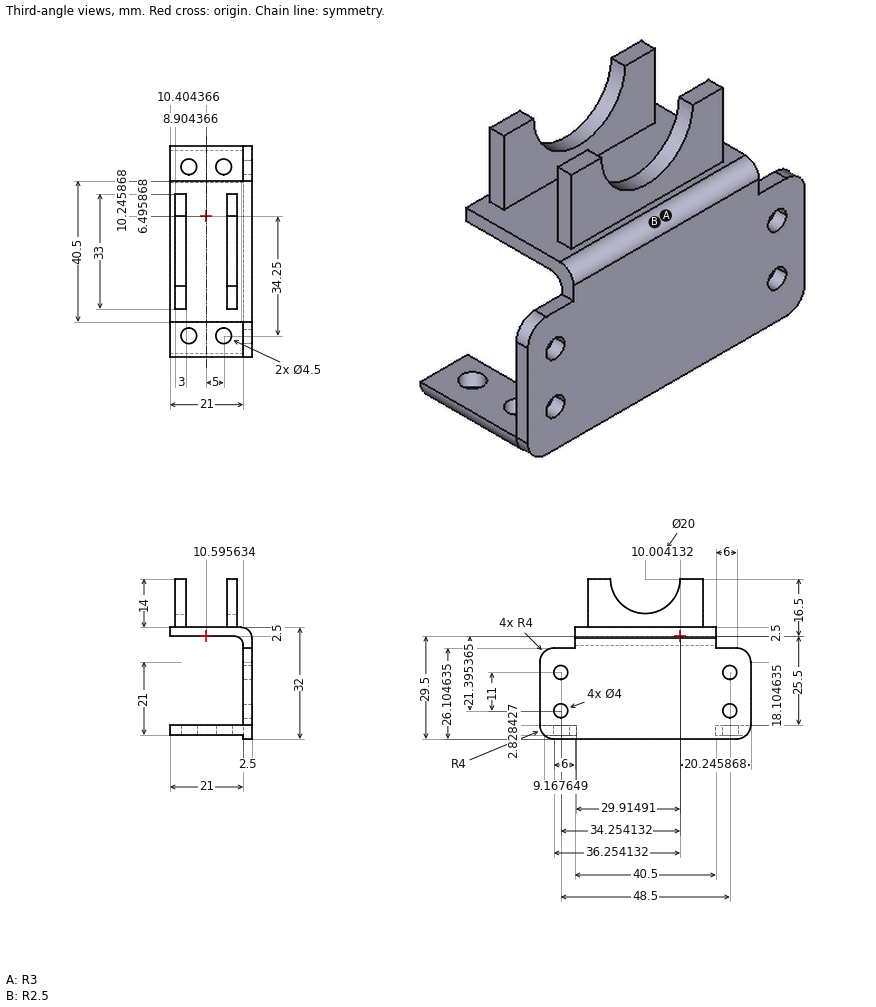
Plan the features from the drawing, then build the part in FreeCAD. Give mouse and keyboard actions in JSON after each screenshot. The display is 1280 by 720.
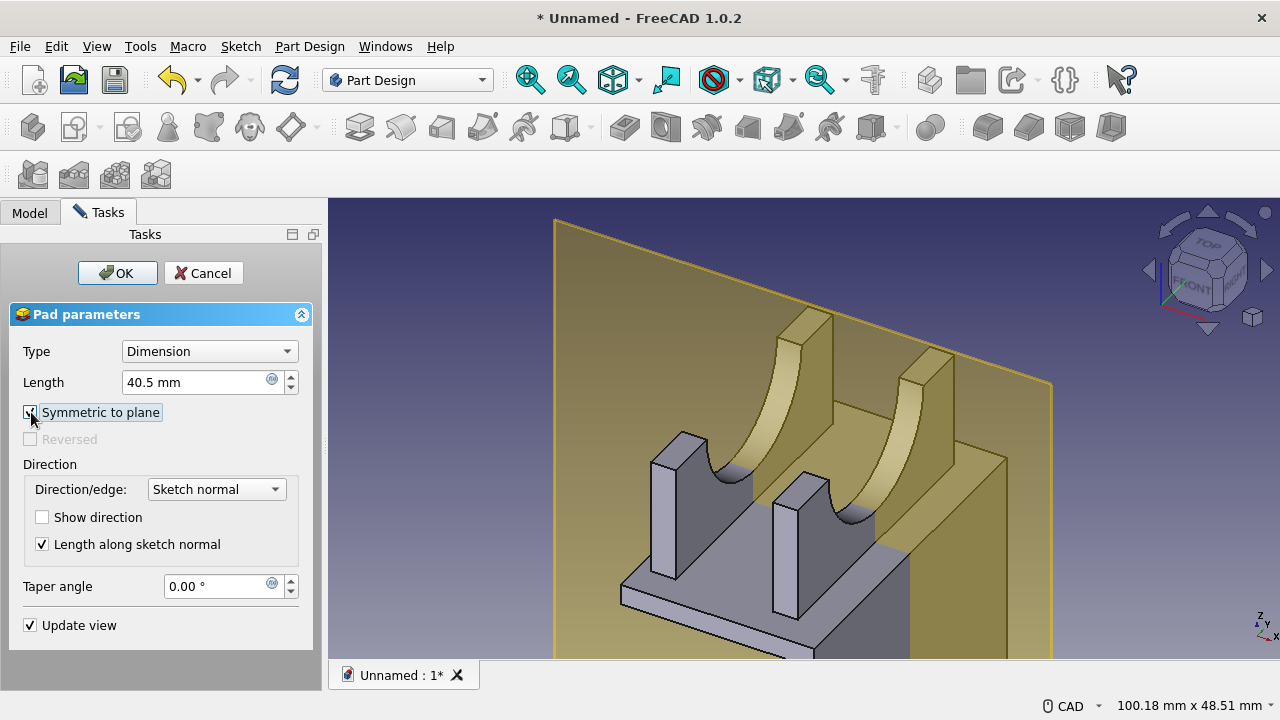
{"action": "left_click", "coordinate": [118, 273]}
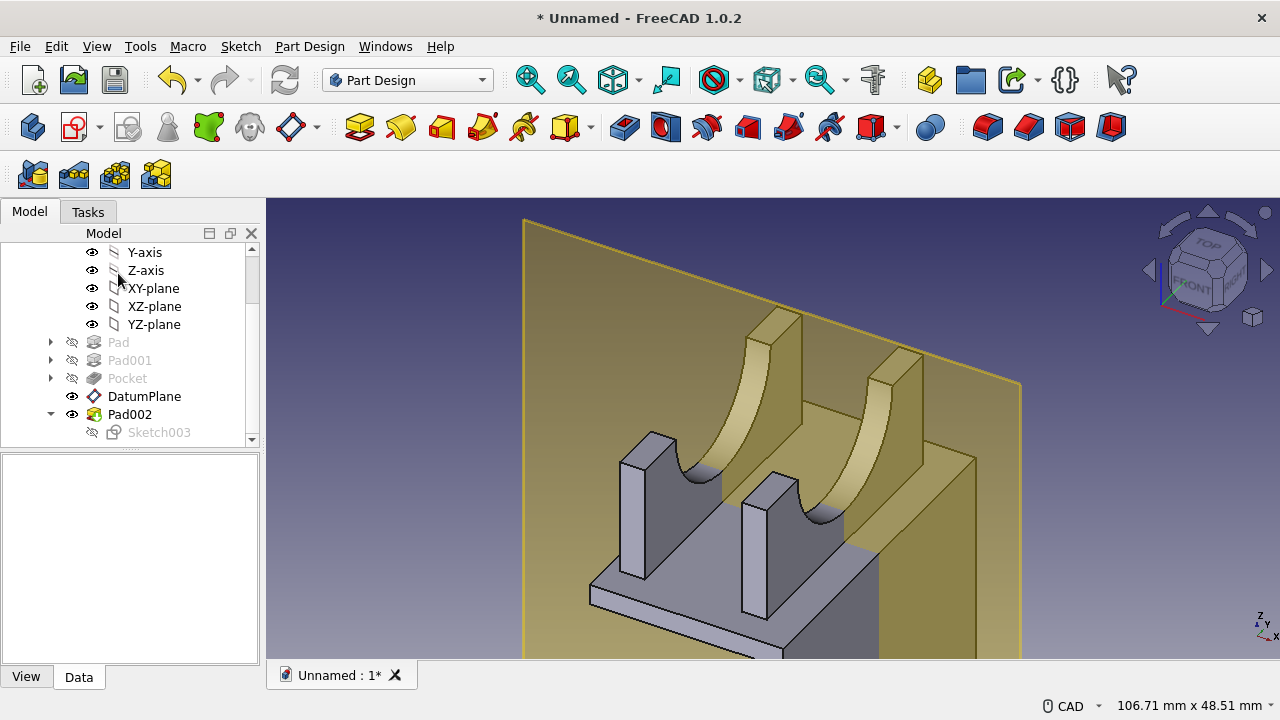
{"action": "left_click", "coordinate": [117, 396]}
{"action": "key", "text": "space"}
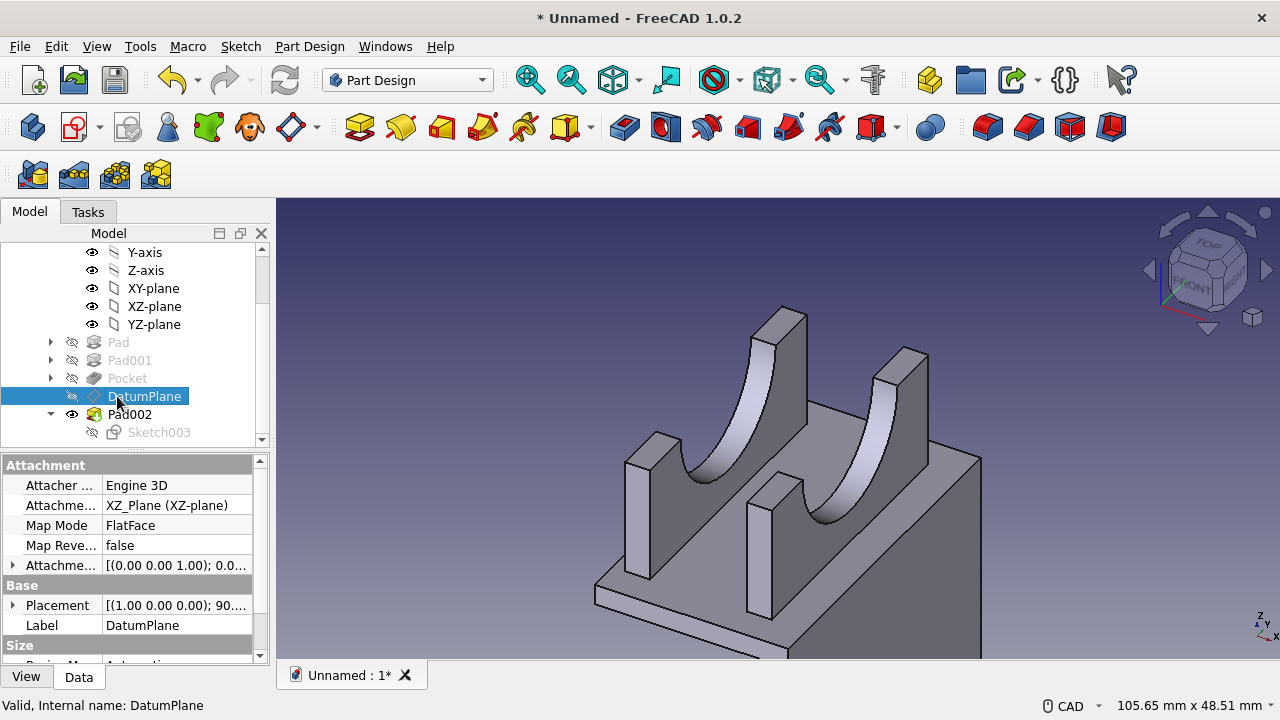
{"action": "key", "text": "v f"}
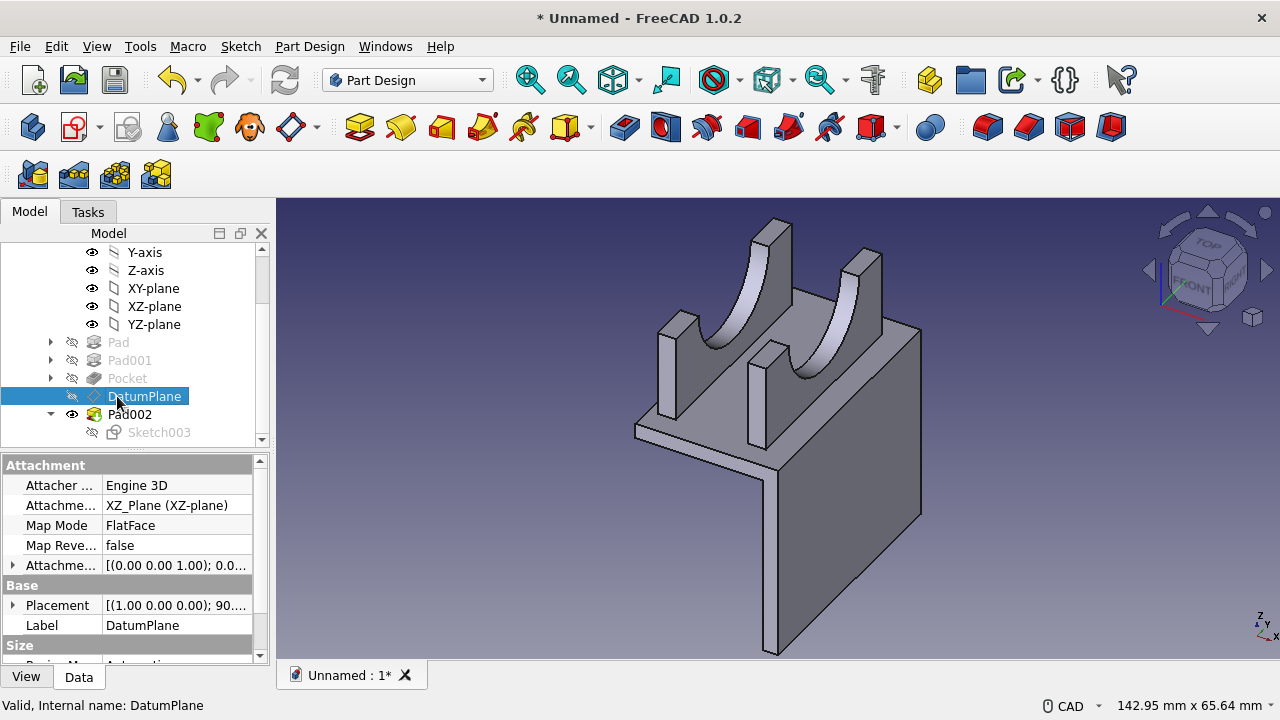
{"action": "left_click", "coordinate": [849, 399]}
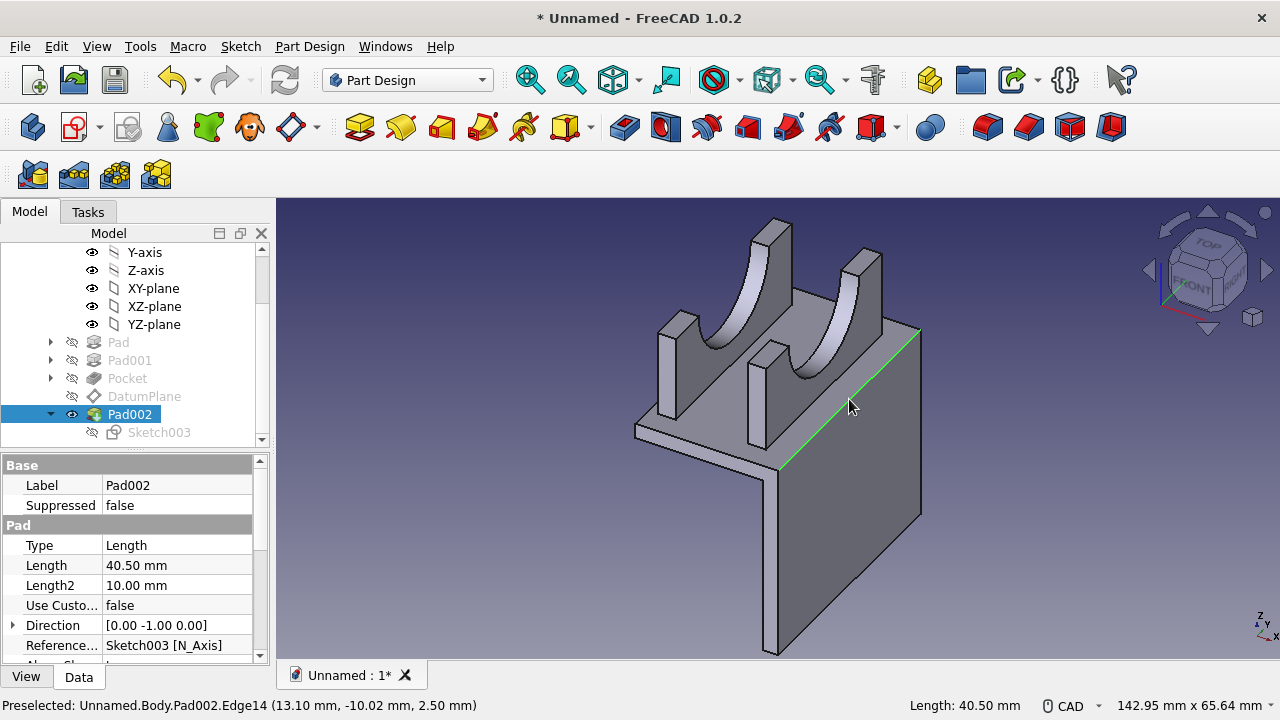
{"action": "left_click", "coordinate": [988, 128]}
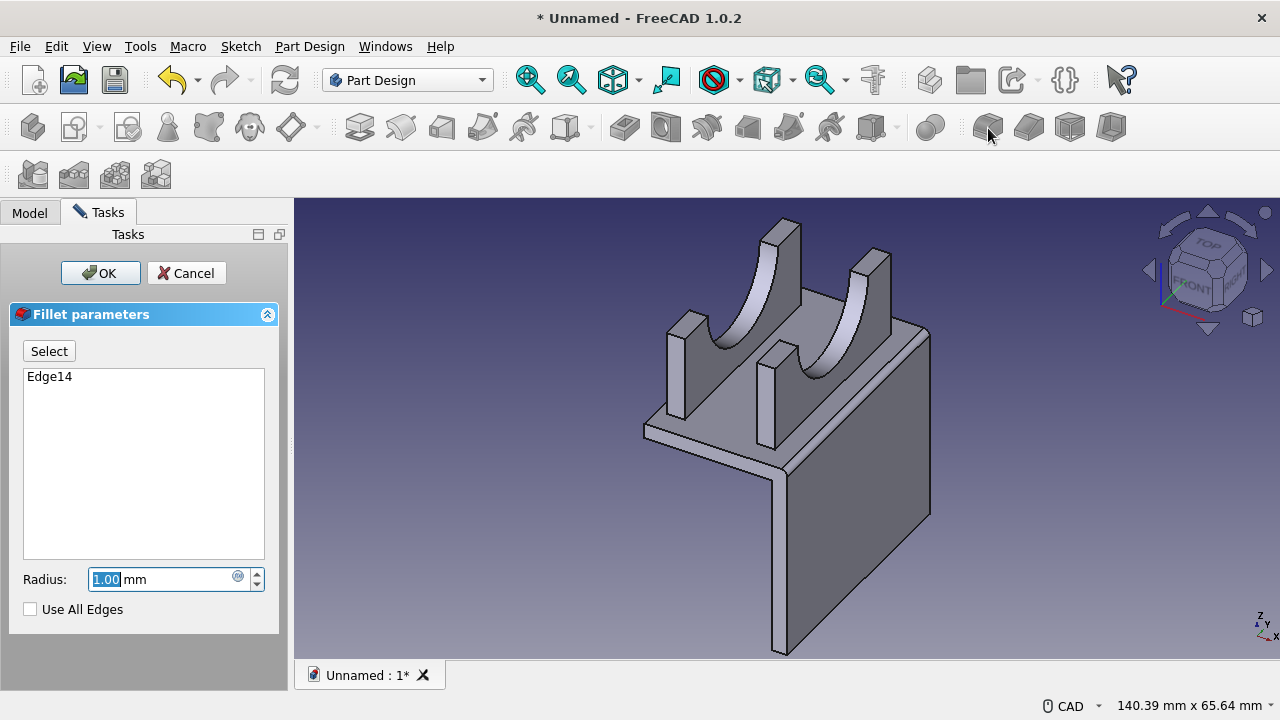
{"action": "type", "text": "3"}
{"action": "key", "text": "Tab"}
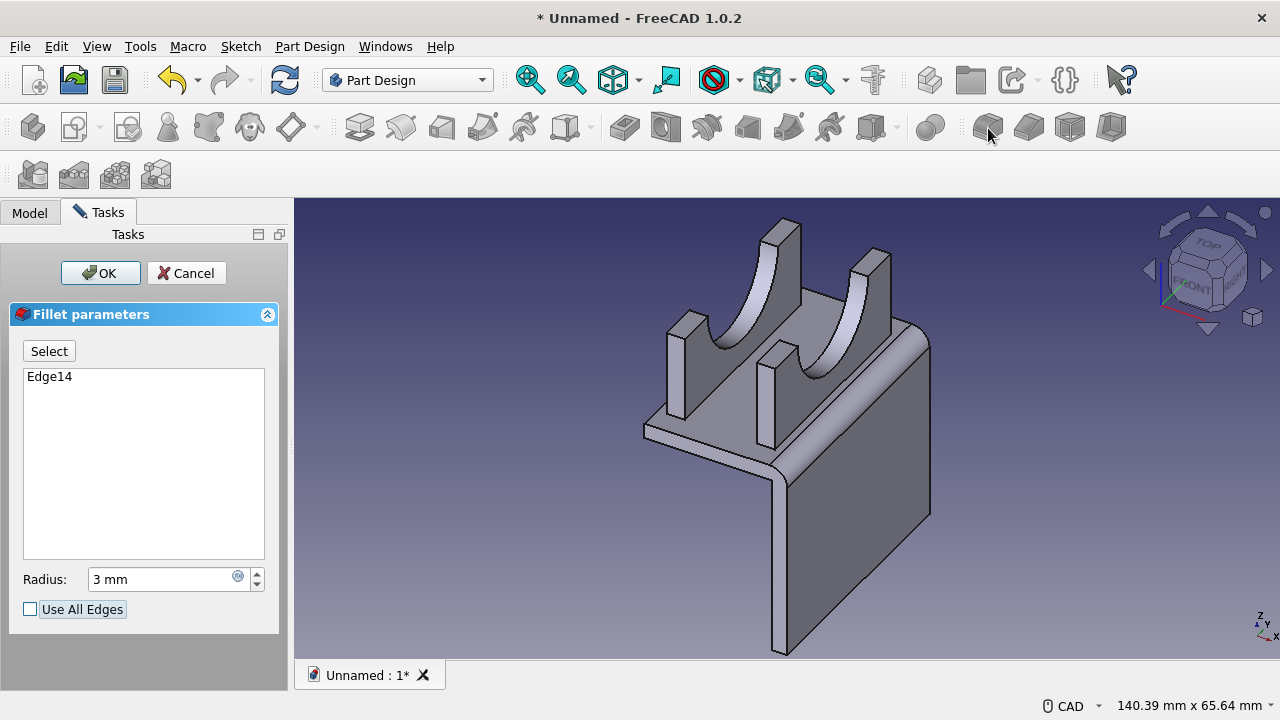
{"action": "left_click", "coordinate": [101, 273]}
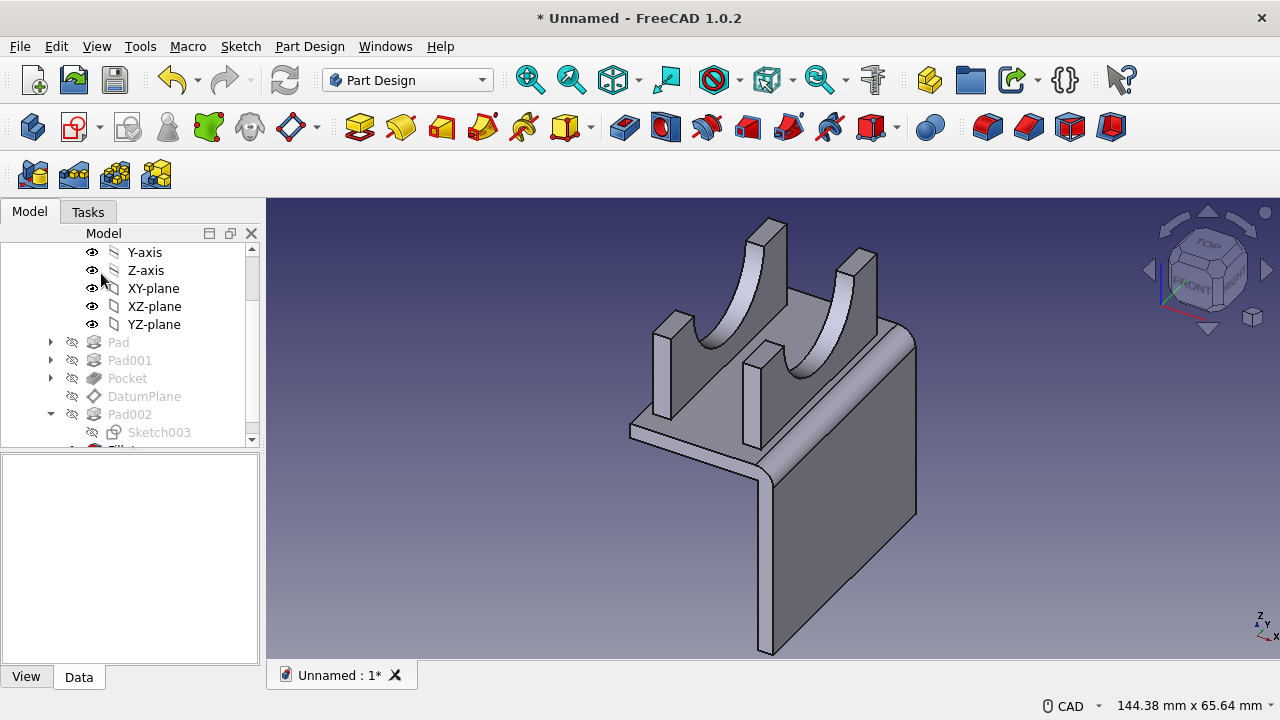
{"action": "key", "text": "0"}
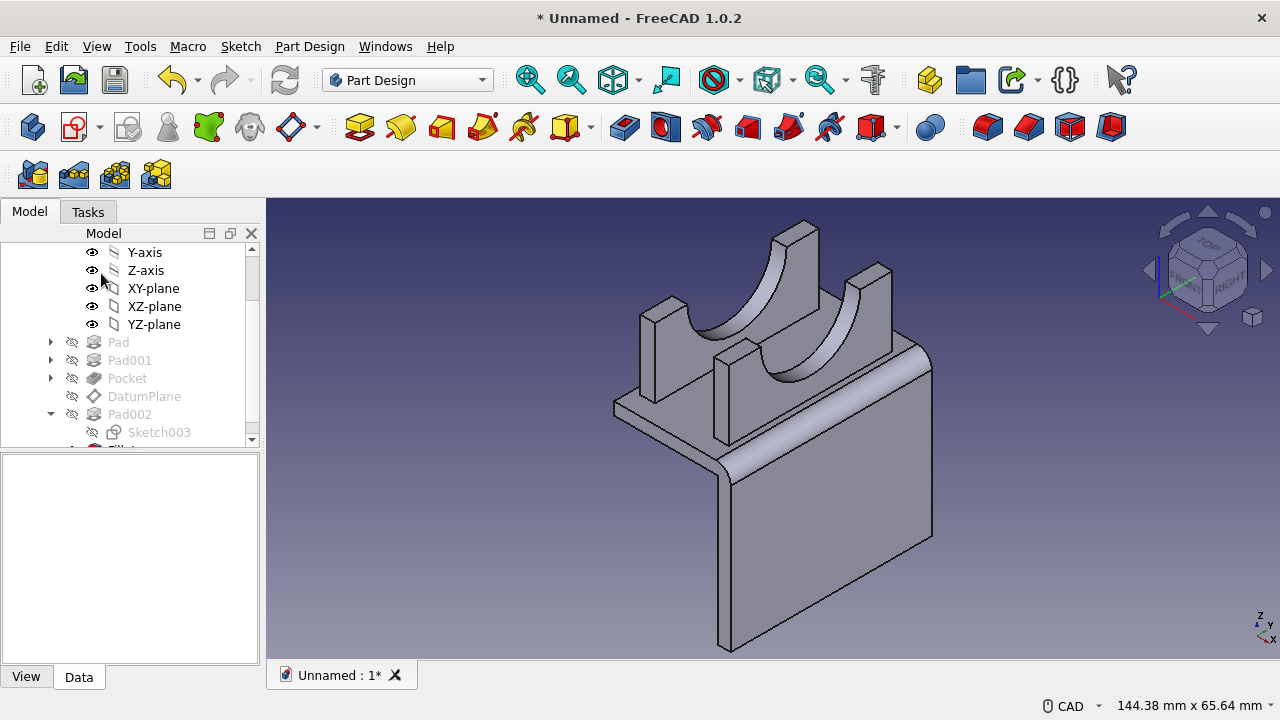
{"action": "key", "text": "2"}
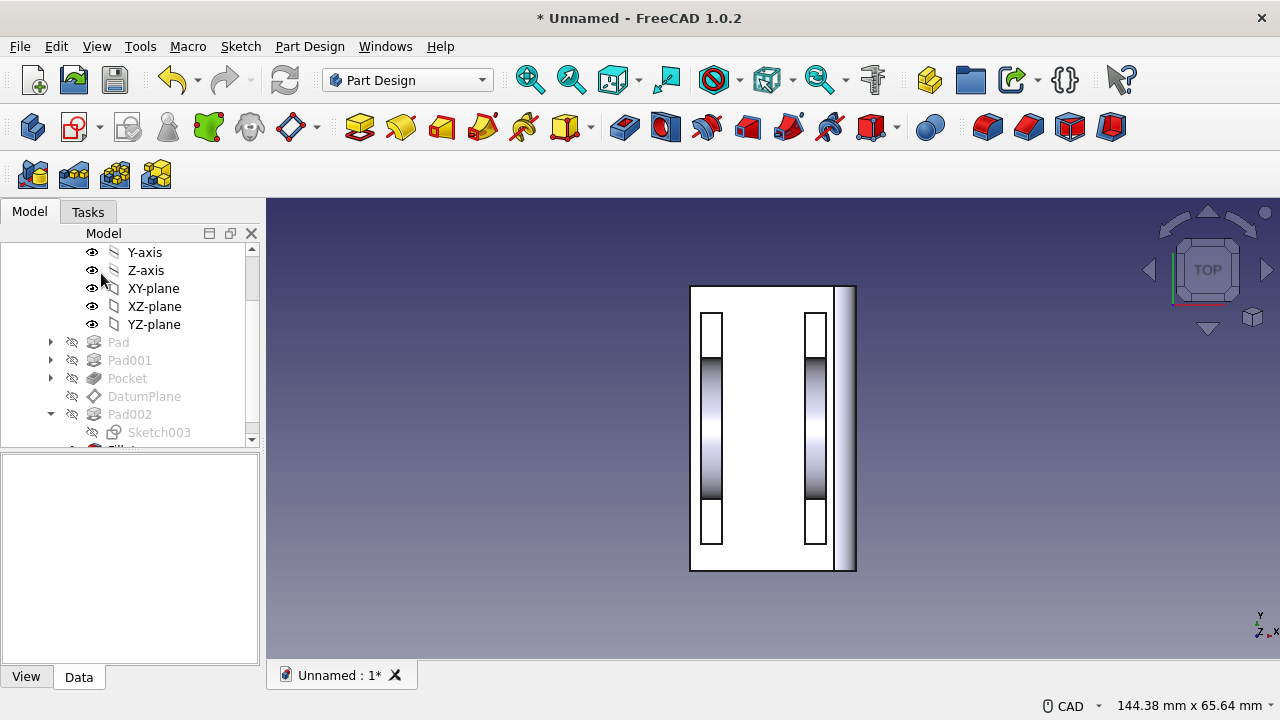
{"action": "key", "text": "1"}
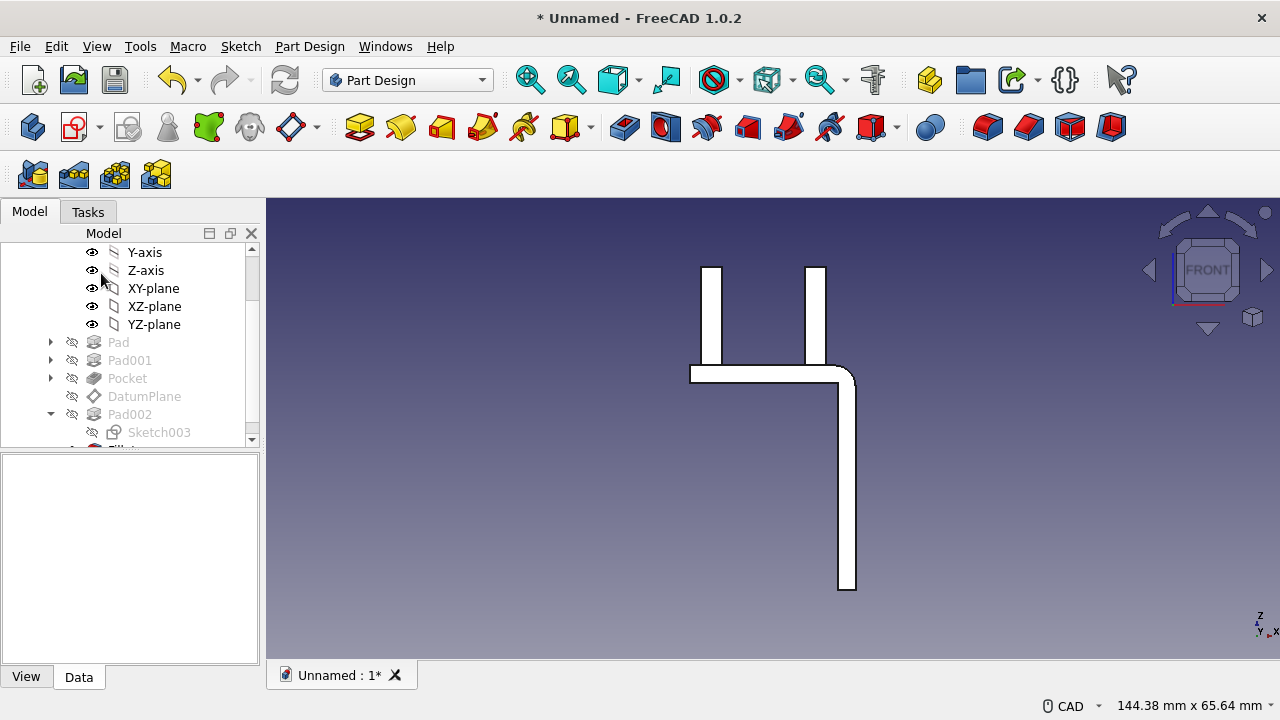
{"action": "key", "text": "3"}